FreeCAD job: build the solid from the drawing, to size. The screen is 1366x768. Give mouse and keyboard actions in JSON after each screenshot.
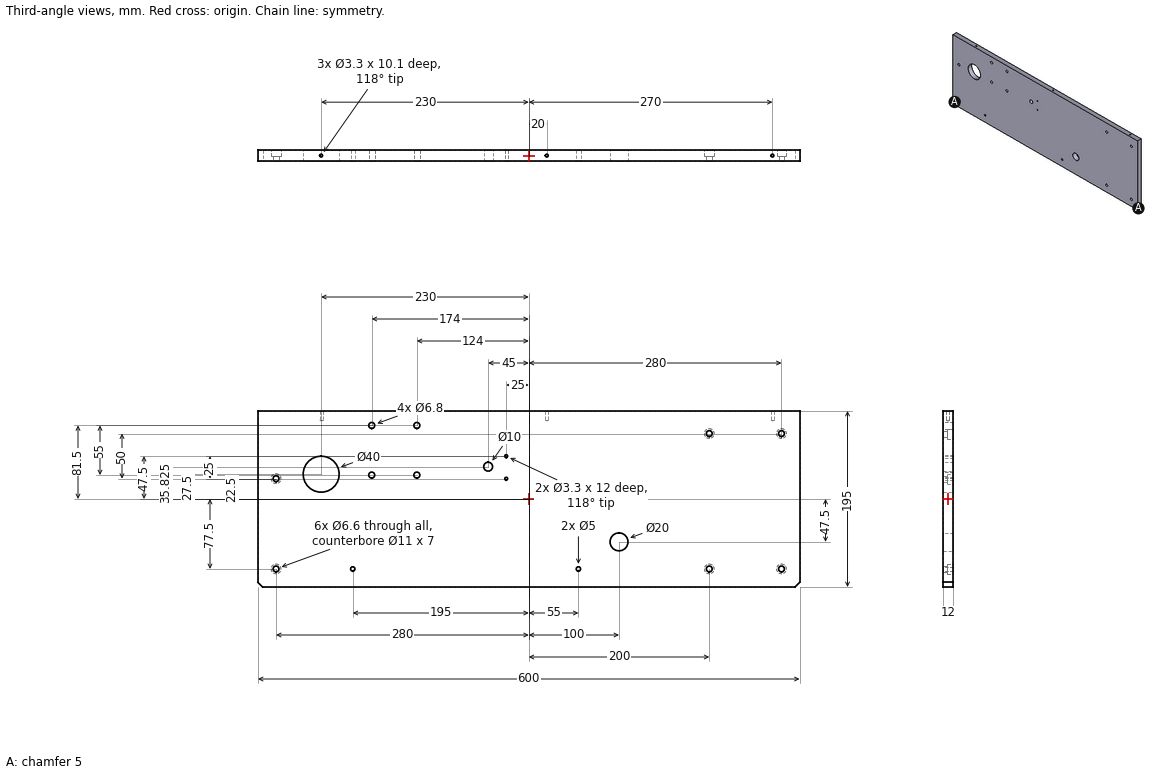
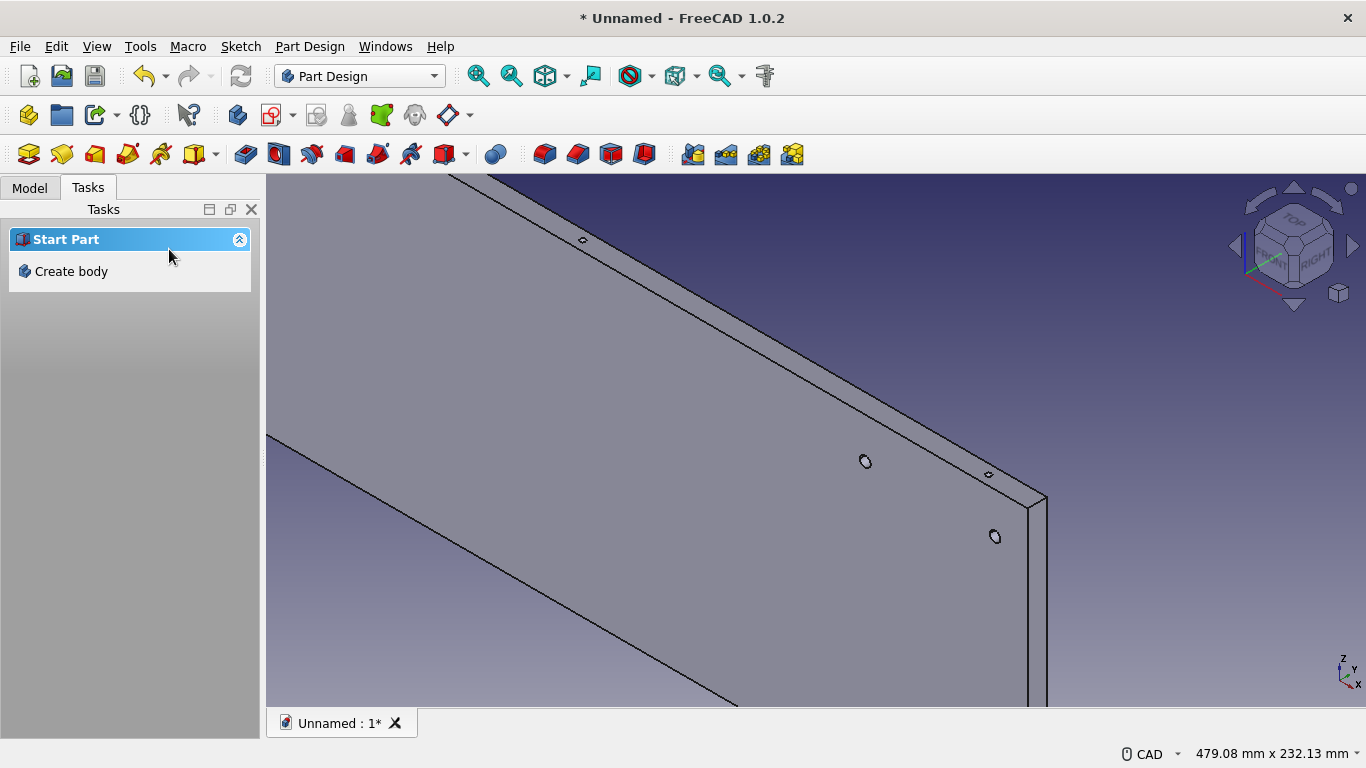
{"action": "left_click", "coordinate": [479, 76]}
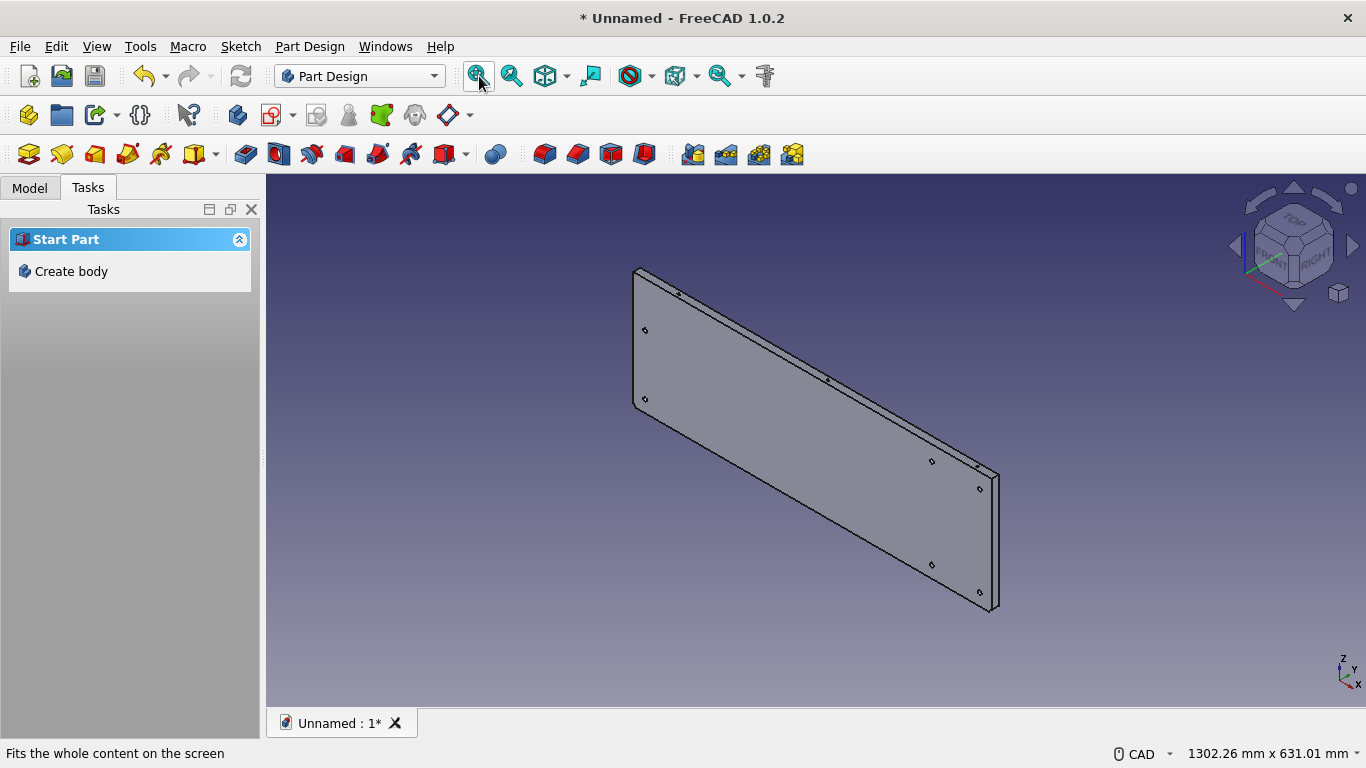
{"action": "key", "text": "4"}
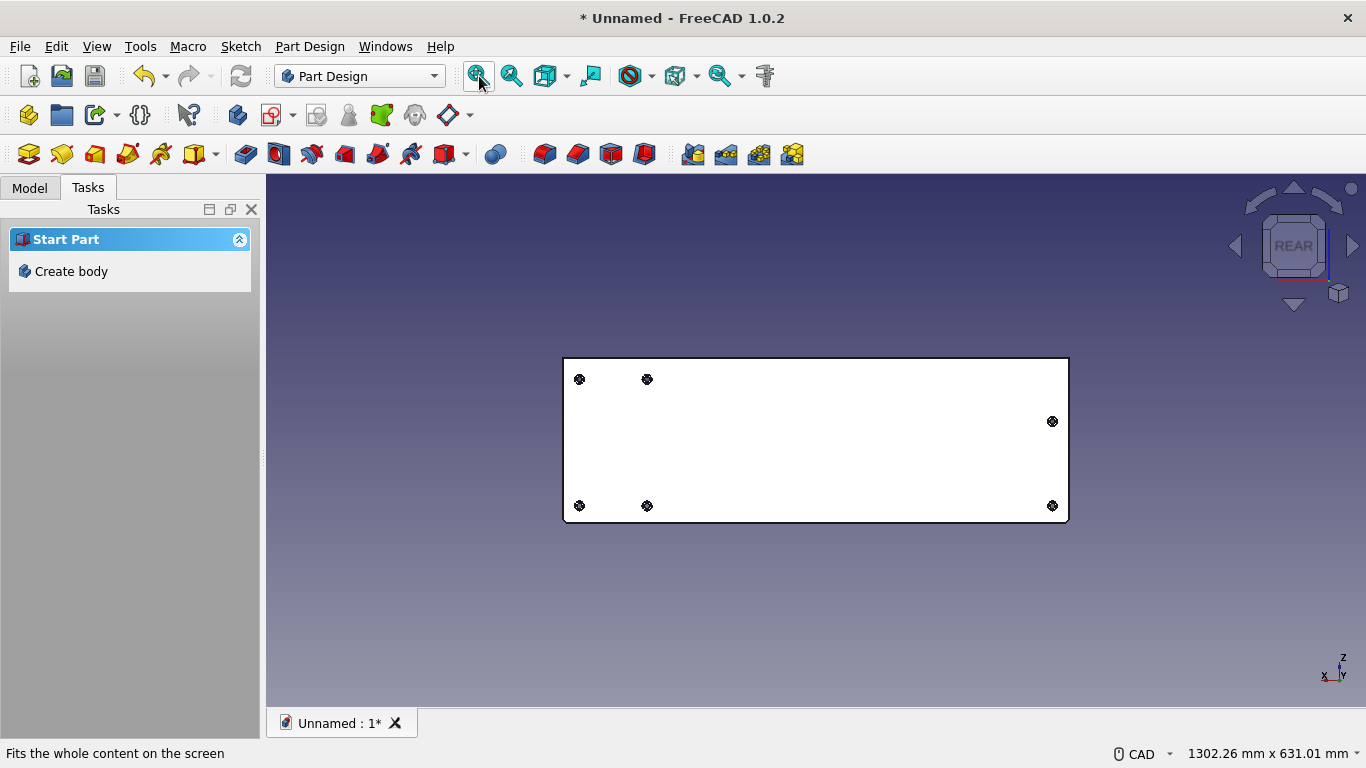
{"action": "left_click", "coordinate": [744, 439]}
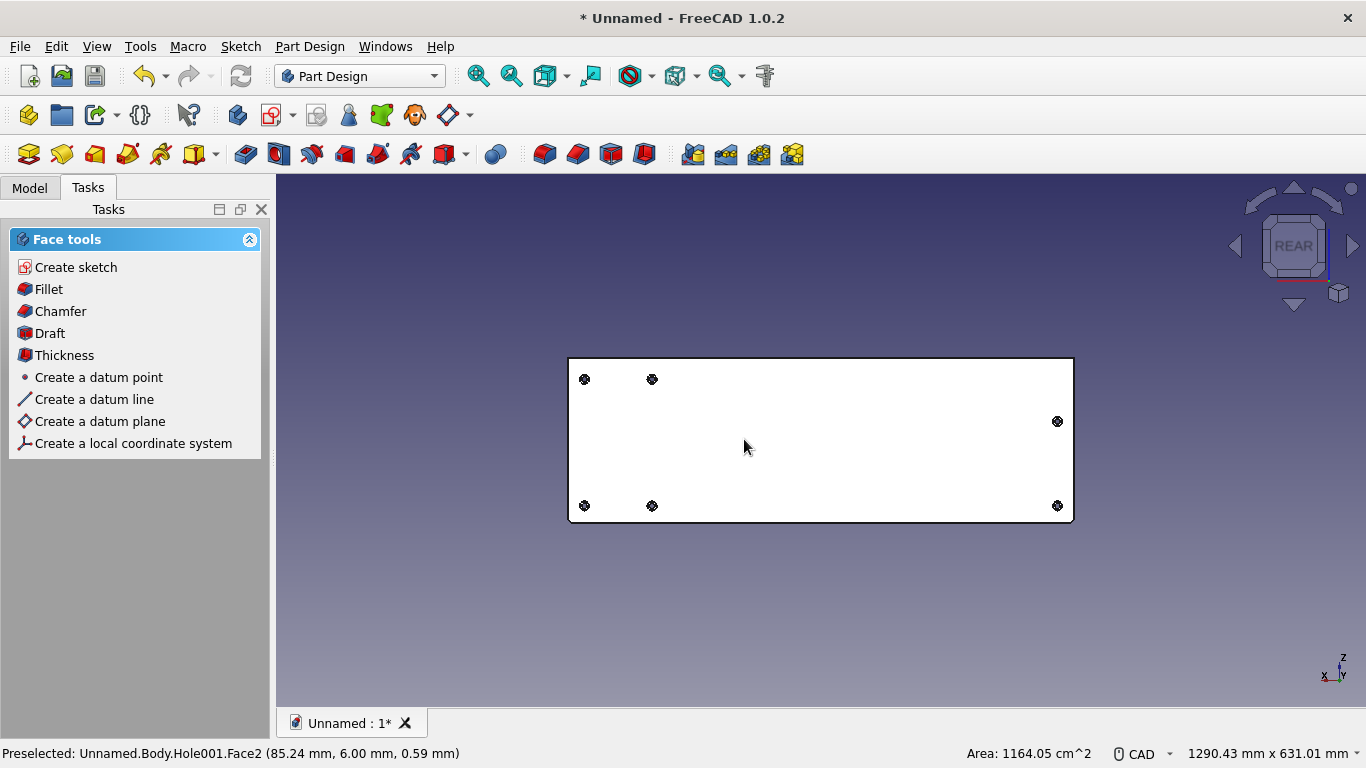
{"action": "left_click", "coordinate": [270, 116]}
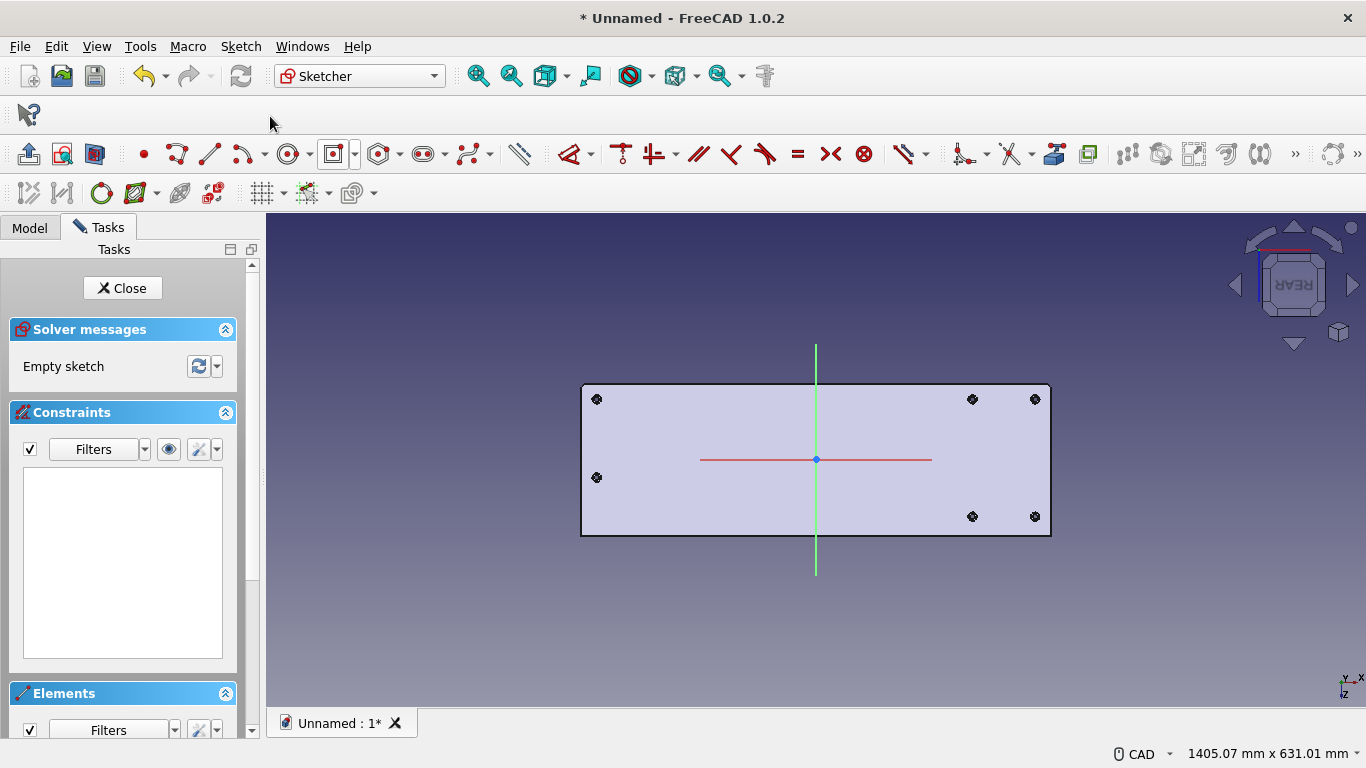
{"action": "scroll", "coordinate": [690, 511], "scroll_direction": "up", "scroll_amount": 9}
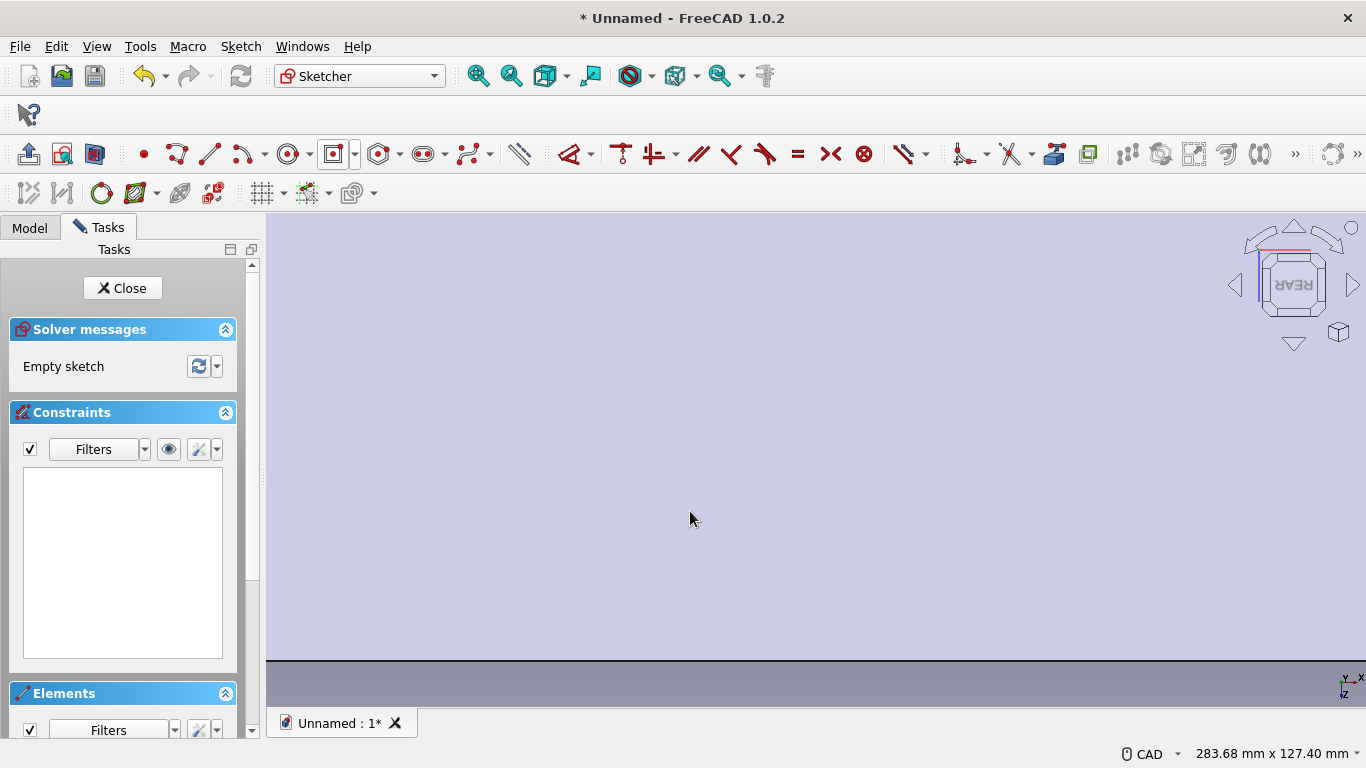
{"action": "left_click", "coordinate": [288, 154]}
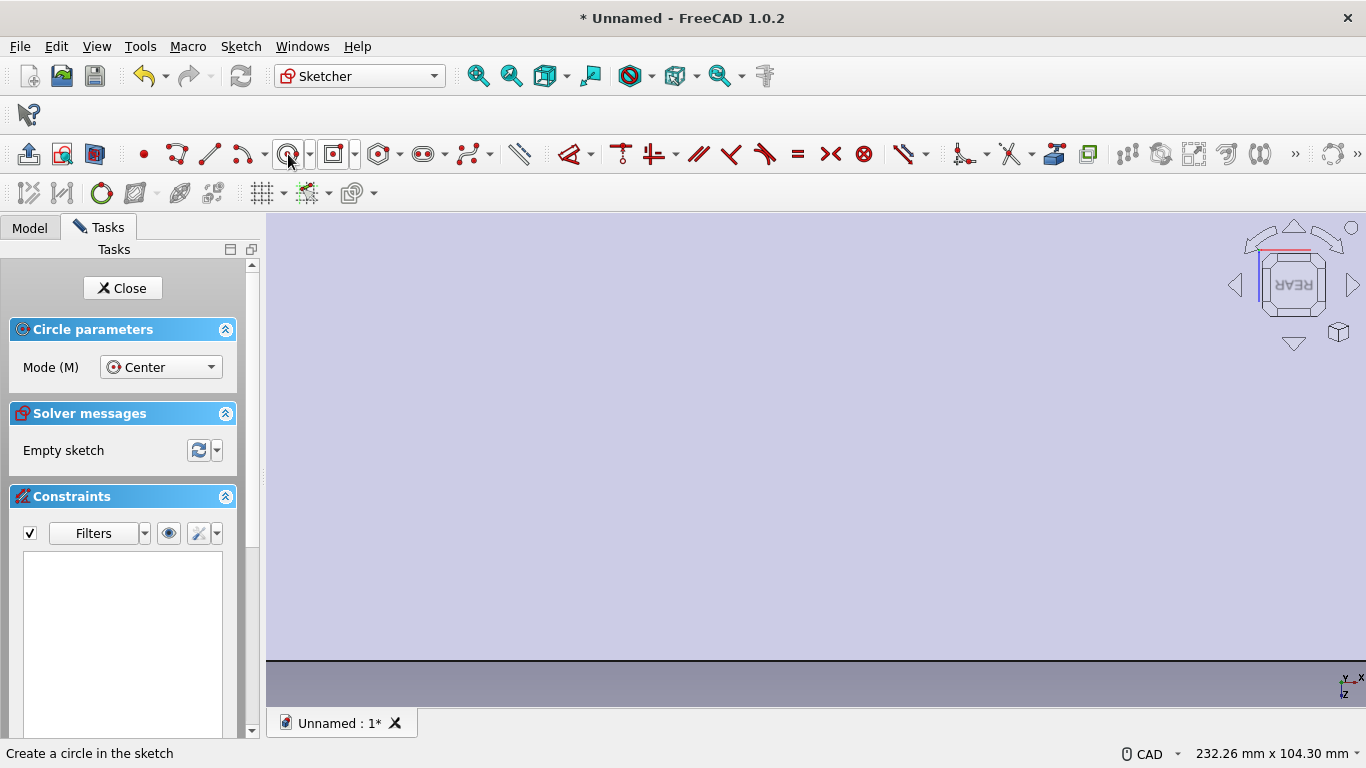
{"action": "scroll", "coordinate": [626, 585], "scroll_direction": "up", "scroll_amount": 2}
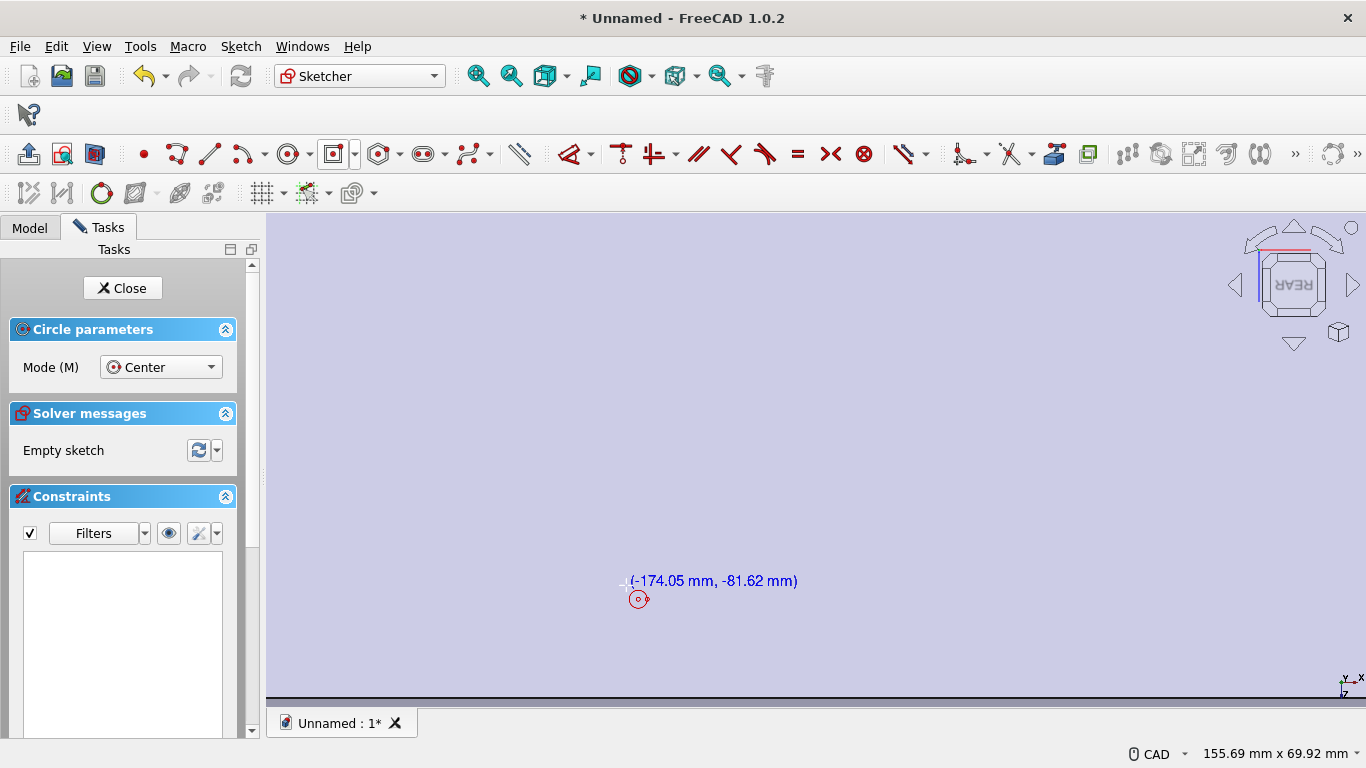
{"action": "left_click", "coordinate": [626, 585]}
{"action": "left_click", "coordinate": [643, 568]}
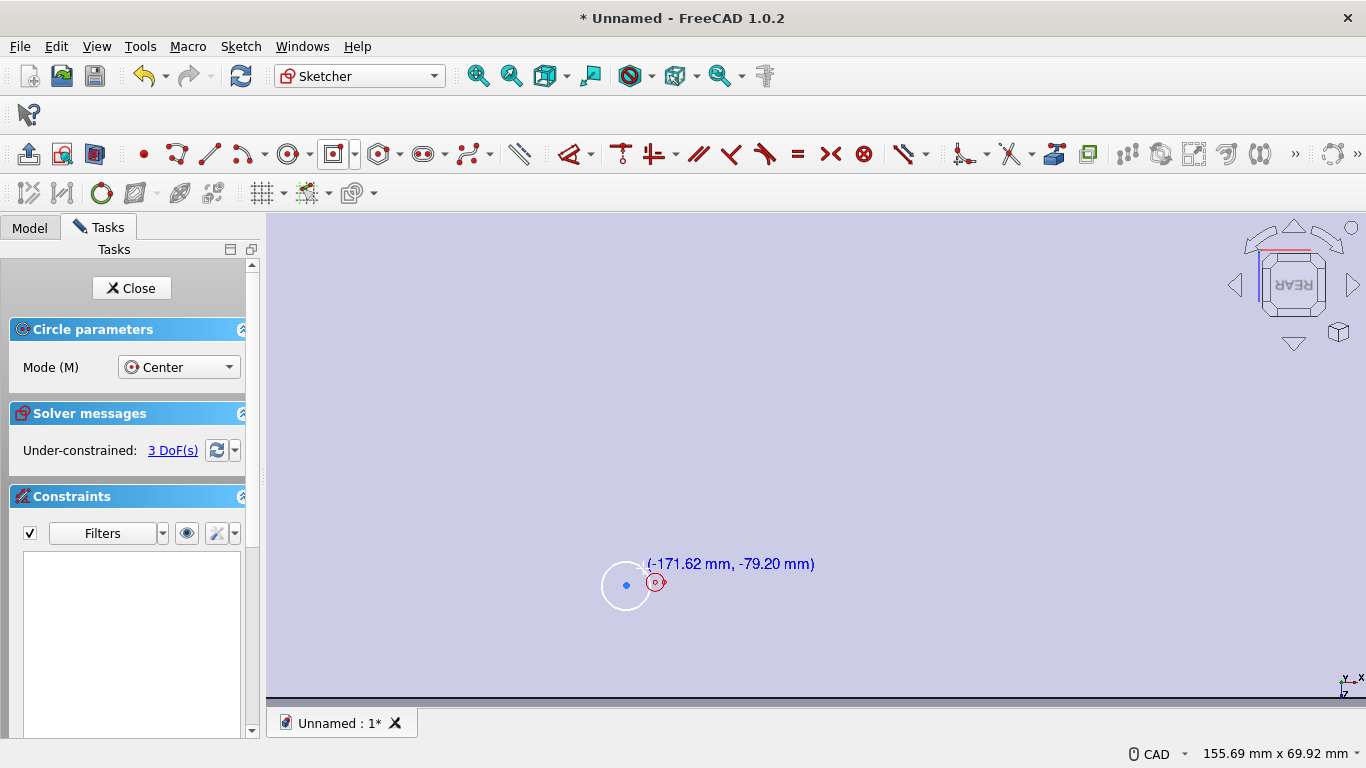
{"action": "left_click", "coordinate": [979, 585]}
{"action": "left_click", "coordinate": [996, 568]}